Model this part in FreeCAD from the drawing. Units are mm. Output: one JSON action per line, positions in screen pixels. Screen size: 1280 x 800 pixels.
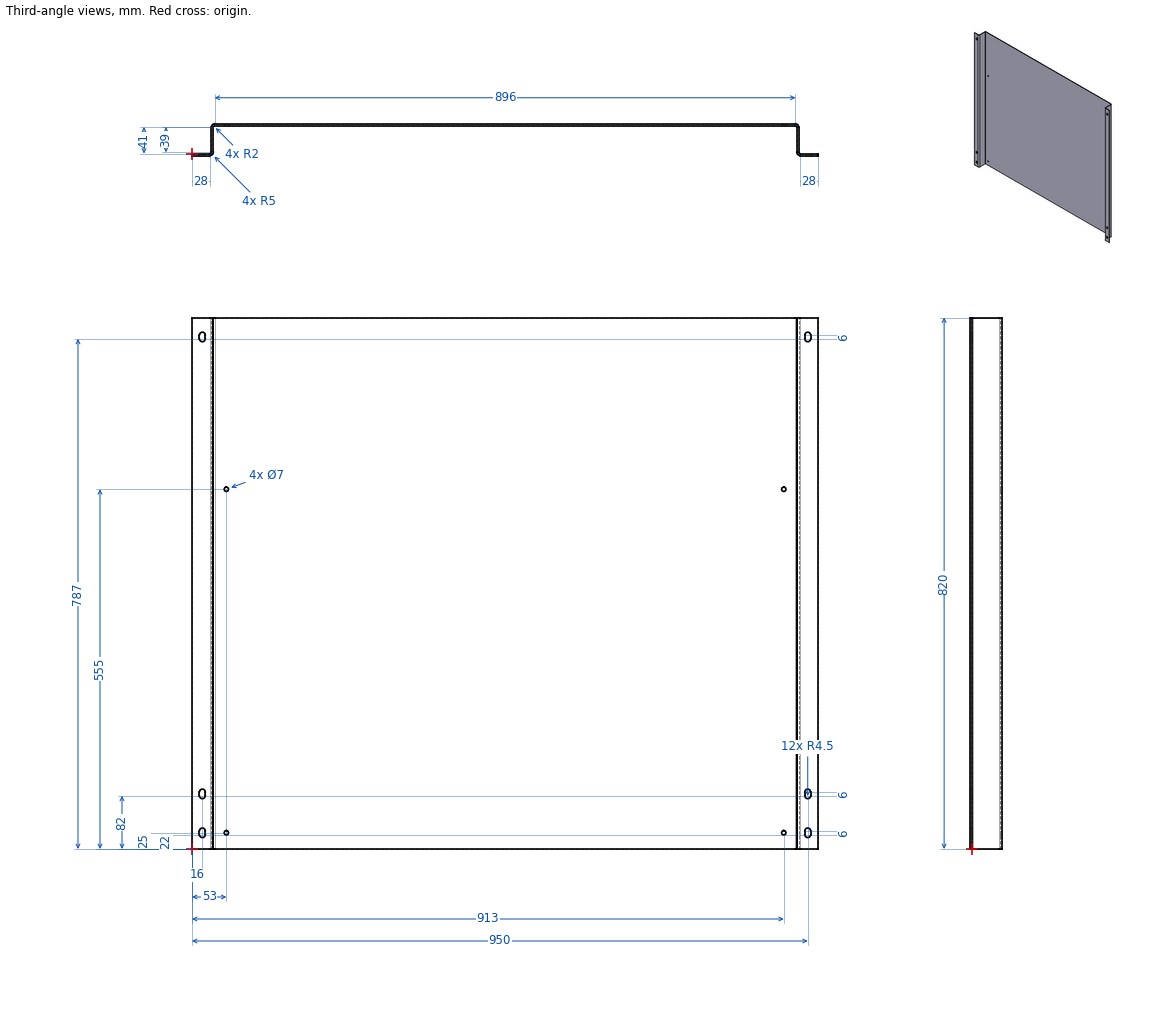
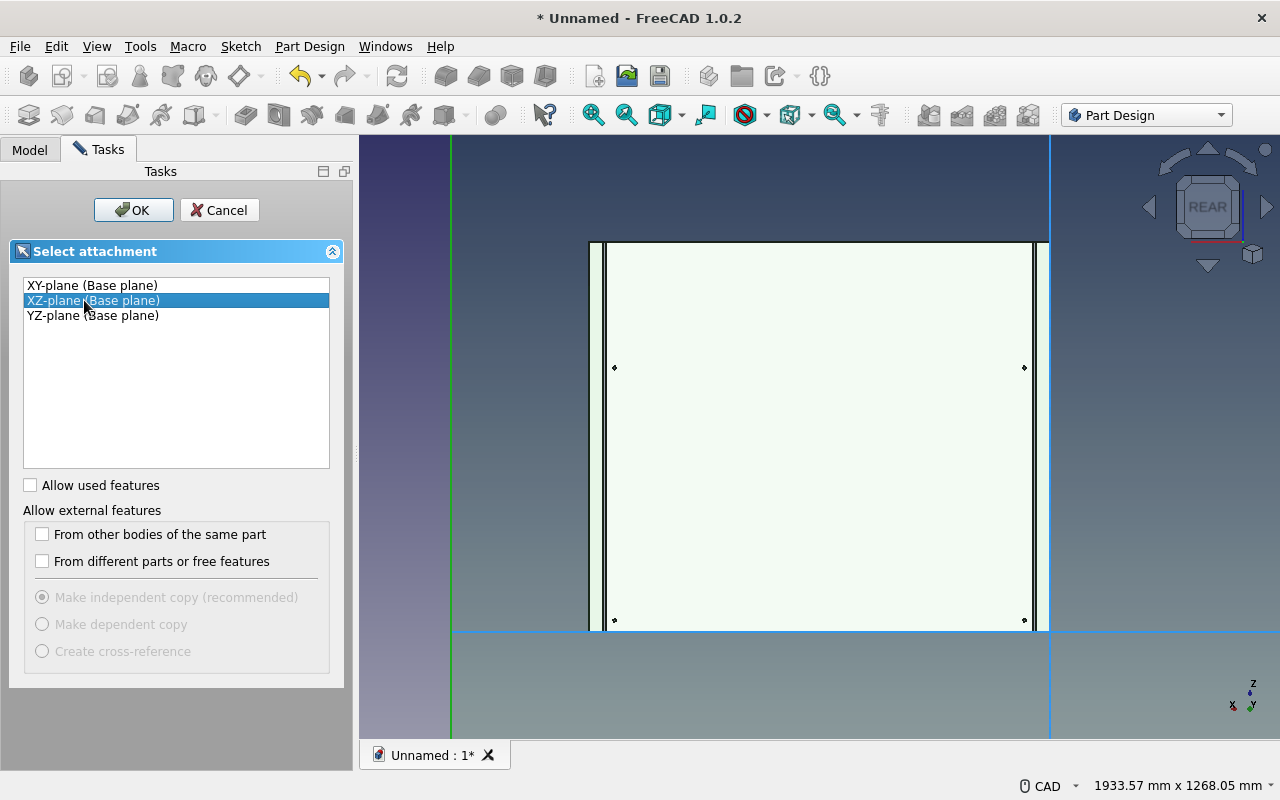
{"action": "left_click", "coordinate": [134, 210]}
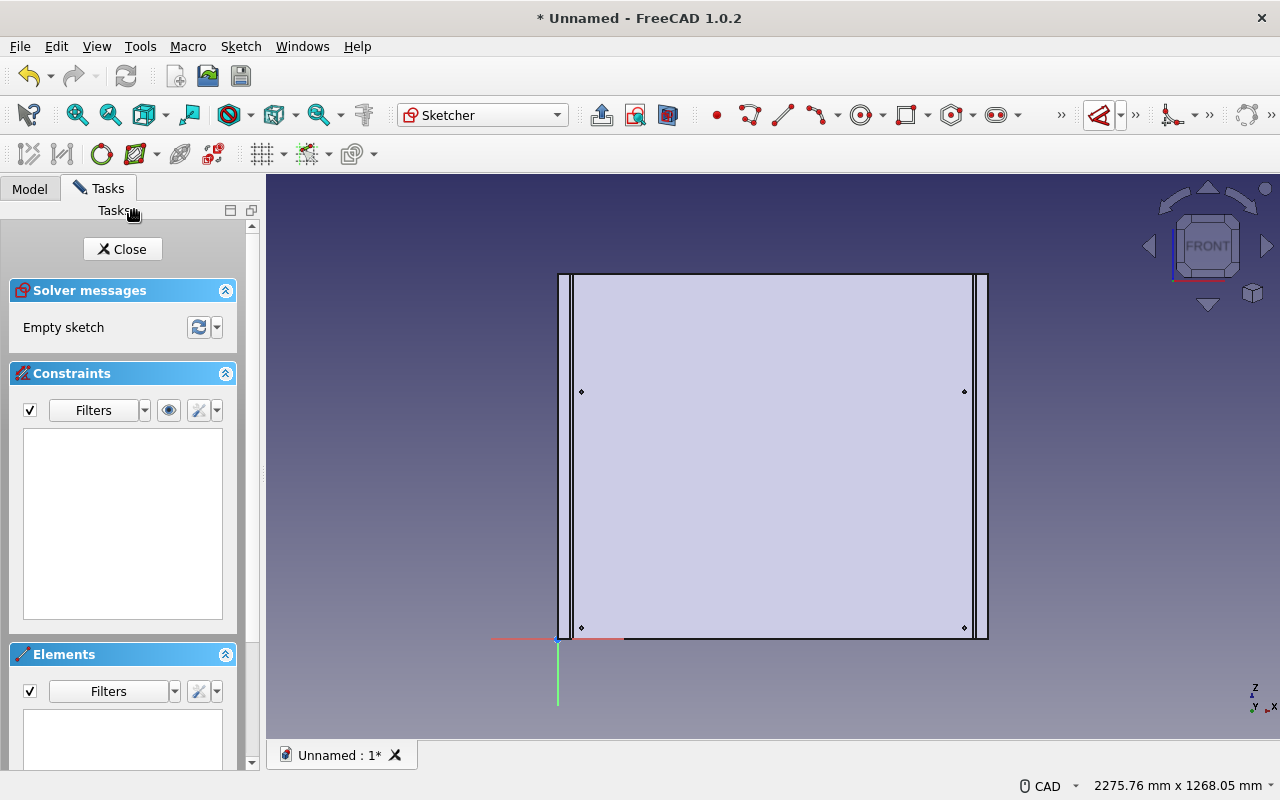
{"action": "left_click", "coordinate": [668, 116]}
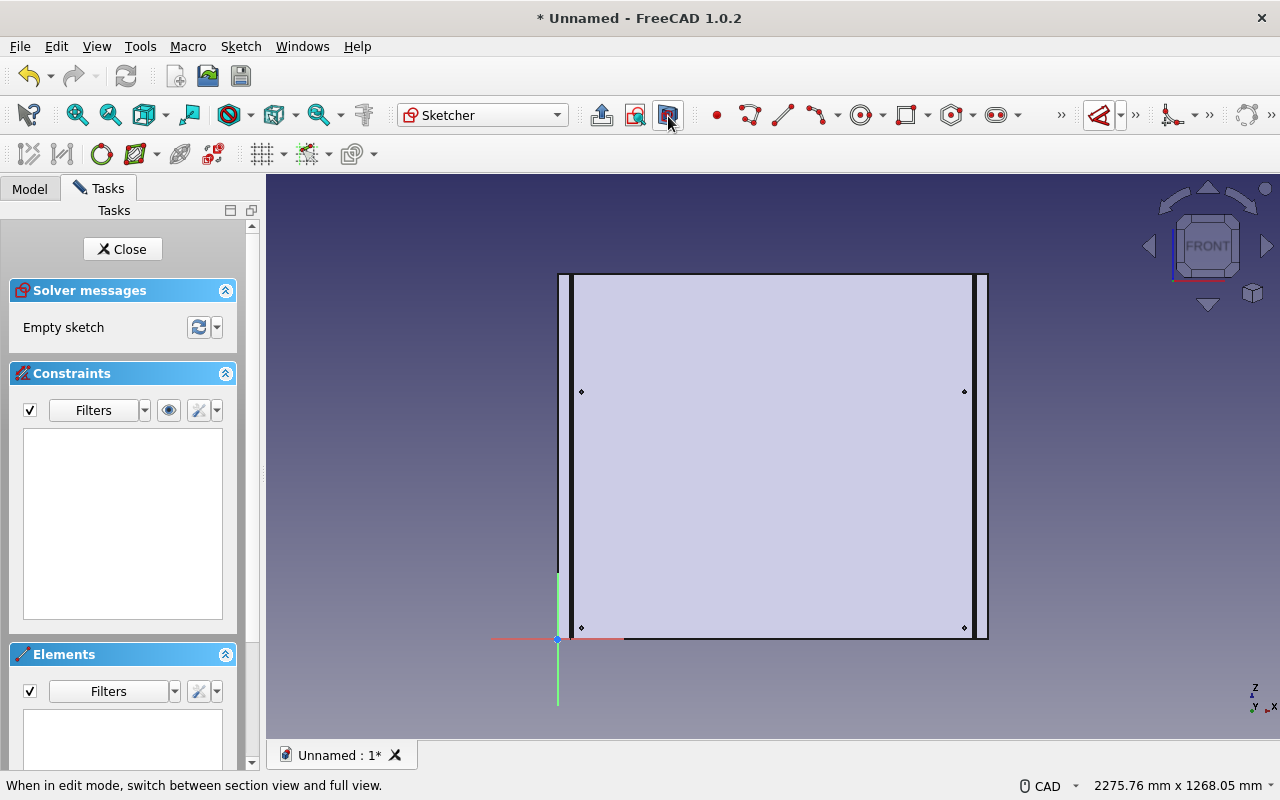
{"action": "key", "text": "g s"}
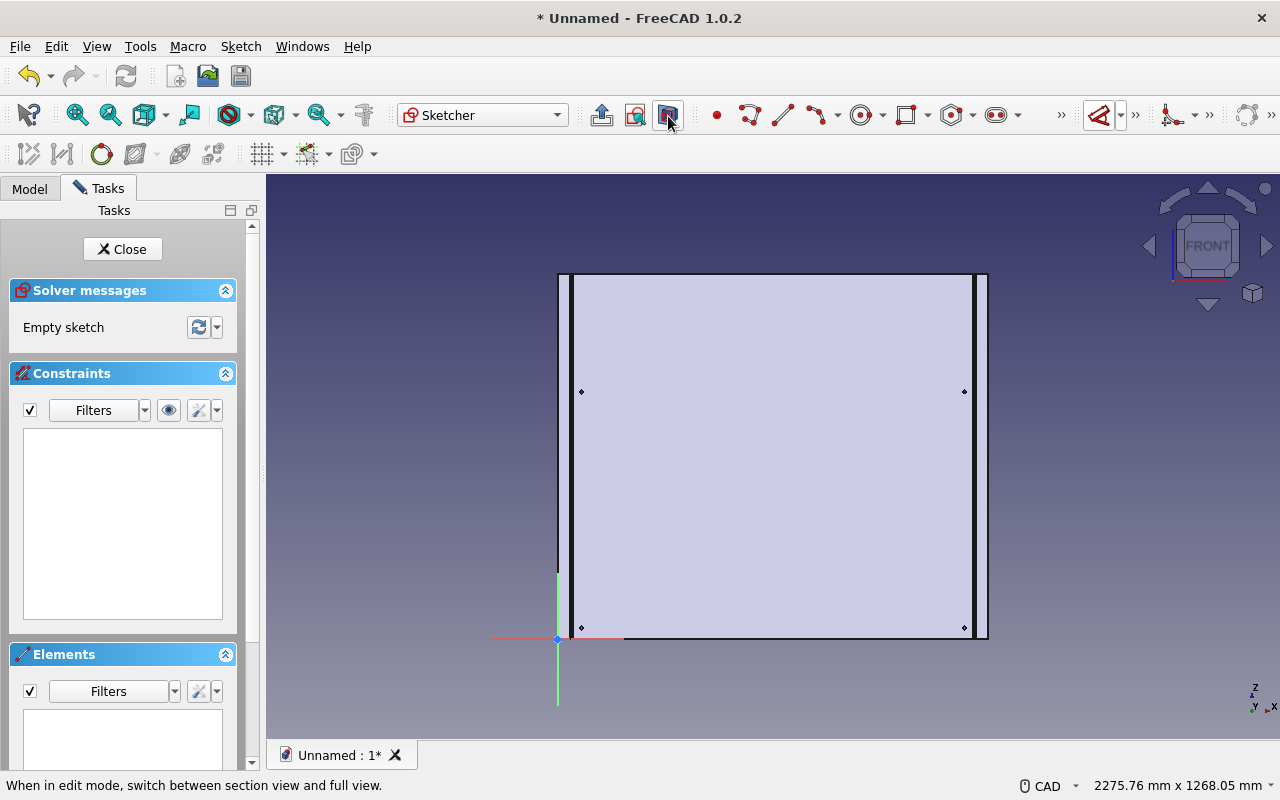
{"action": "scroll", "coordinate": [981, 603], "scroll_direction": "up", "scroll_amount": 13}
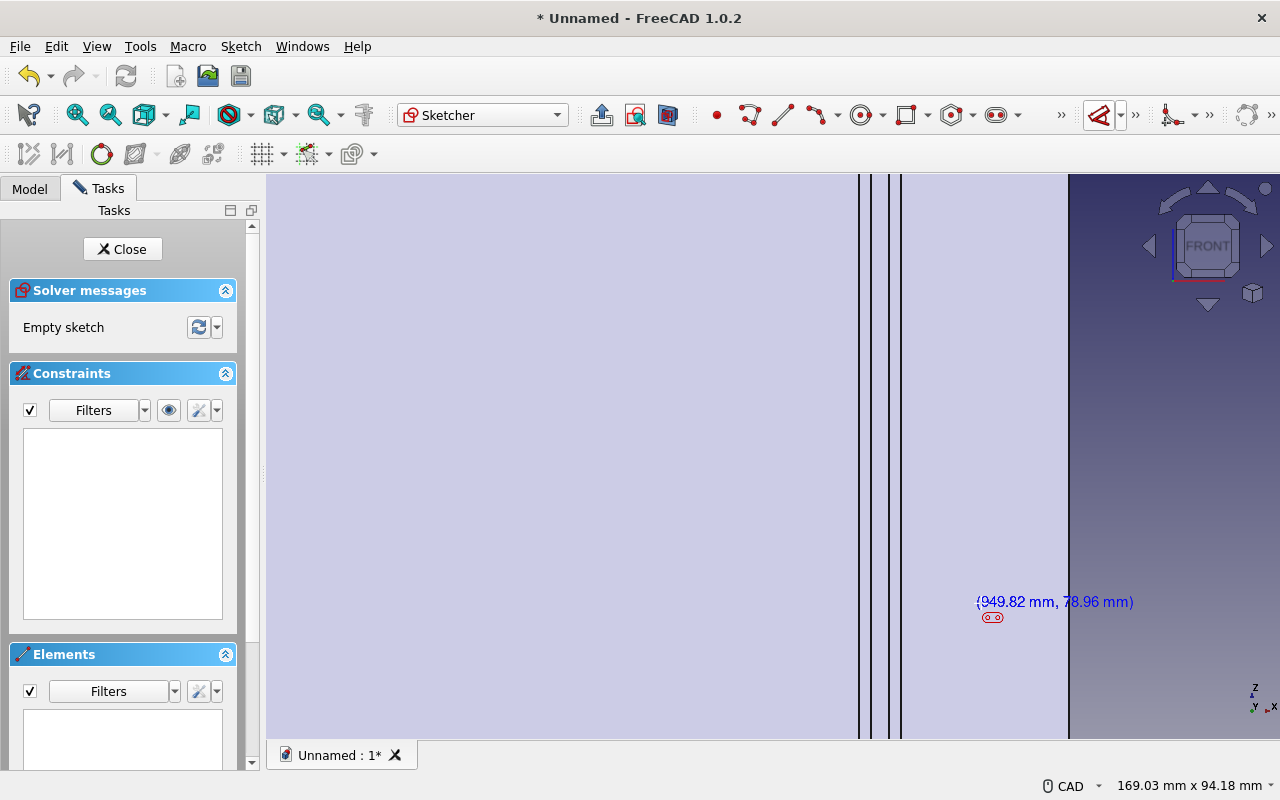
{"action": "scroll", "coordinate": [910, 598], "scroll_direction": "down", "scroll_amount": 13}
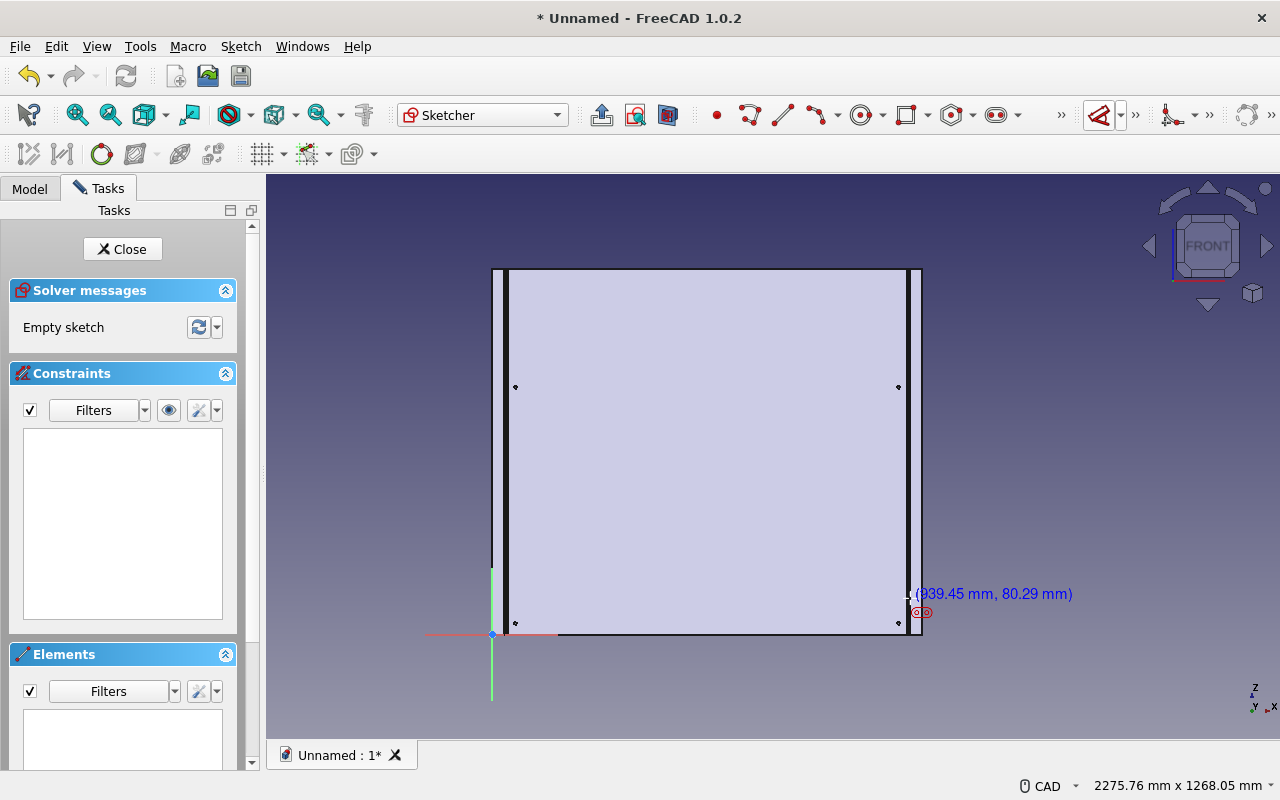
{"action": "left_click", "coordinate": [915, 598]}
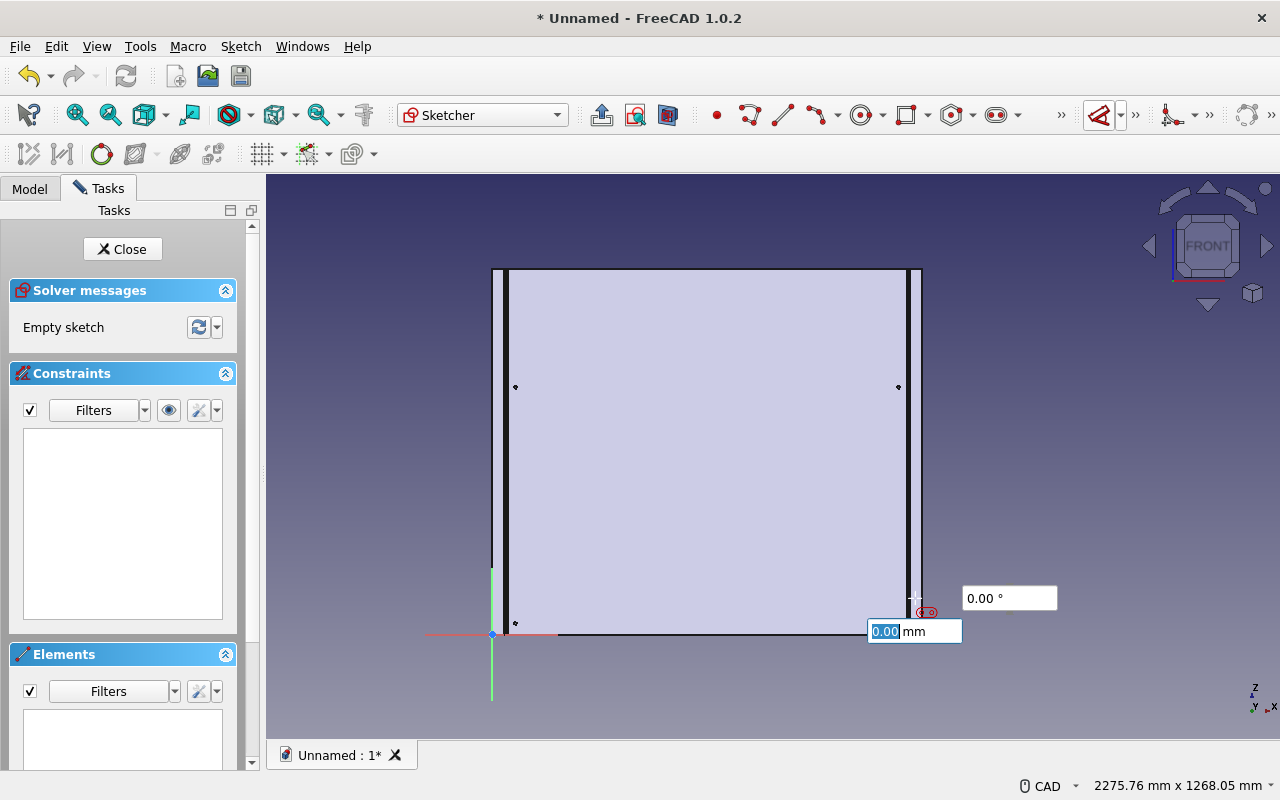
{"action": "scroll", "coordinate": [915, 595], "scroll_direction": "up", "scroll_amount": 9}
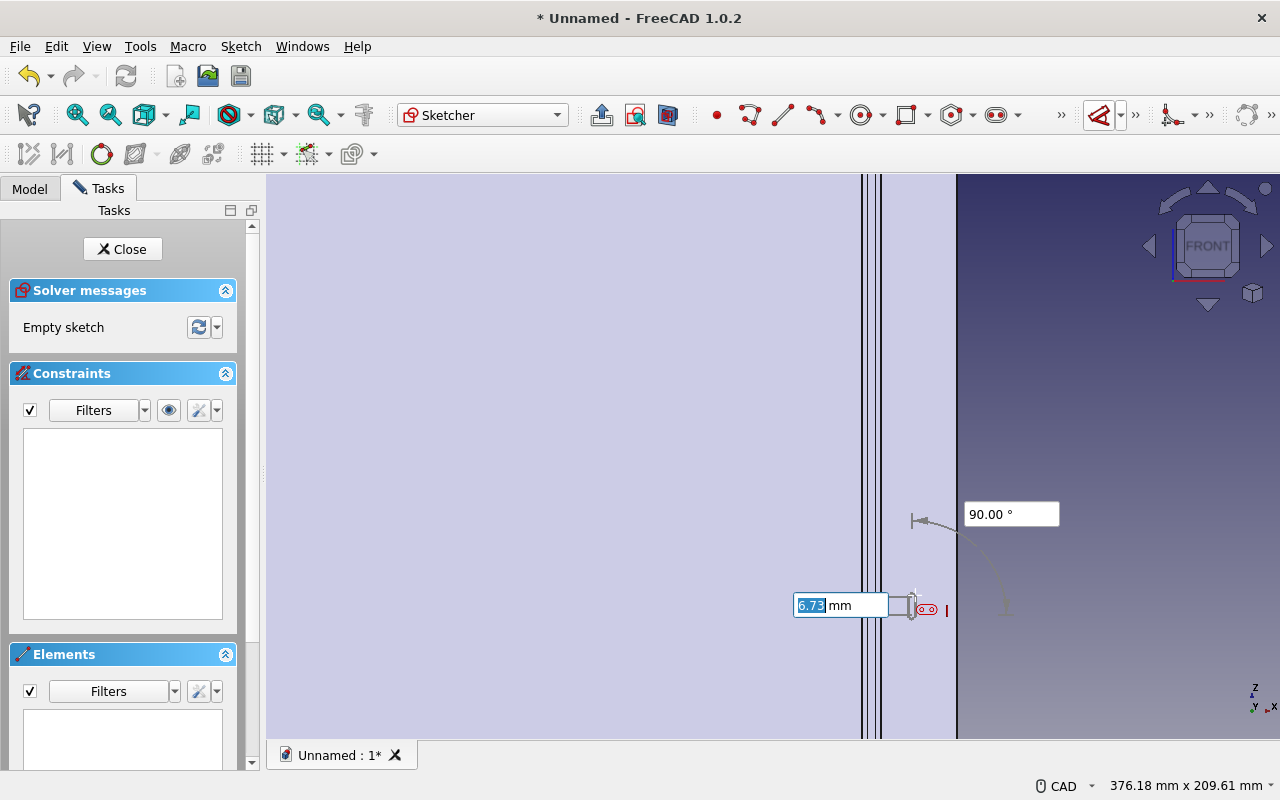
{"action": "left_click", "coordinate": [912, 593]}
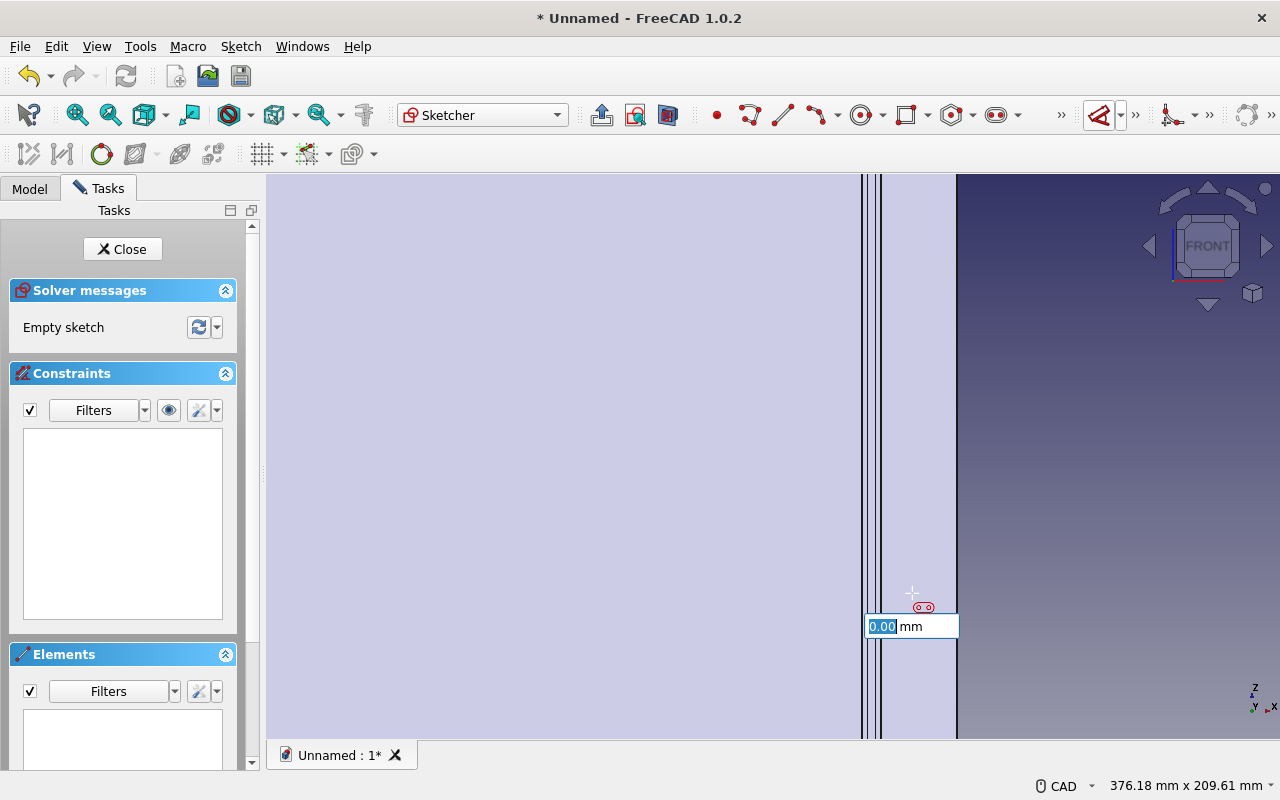
{"action": "scroll", "coordinate": [926, 601], "scroll_direction": "up", "scroll_amount": 2}